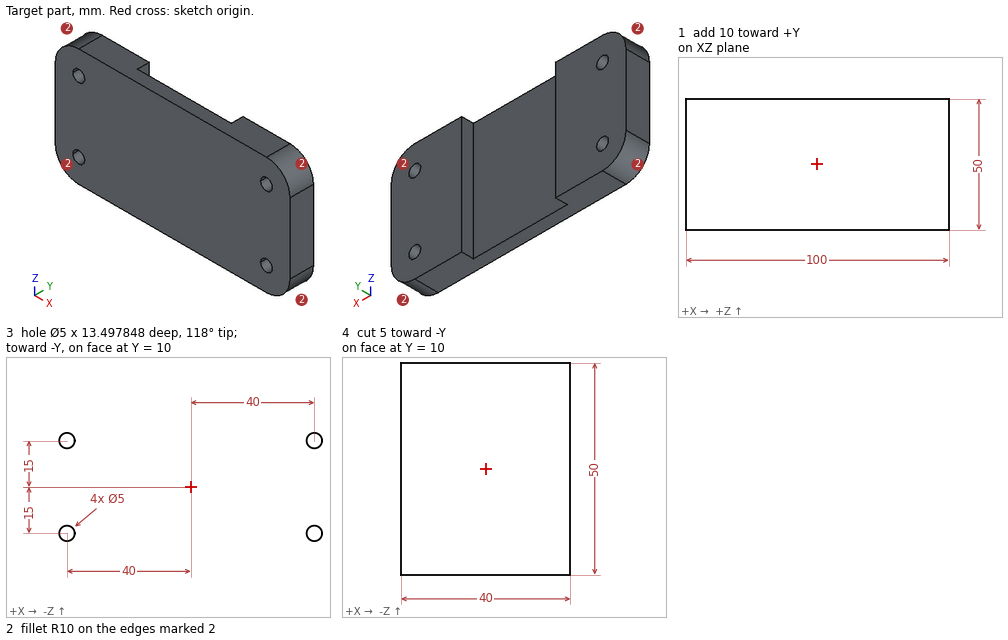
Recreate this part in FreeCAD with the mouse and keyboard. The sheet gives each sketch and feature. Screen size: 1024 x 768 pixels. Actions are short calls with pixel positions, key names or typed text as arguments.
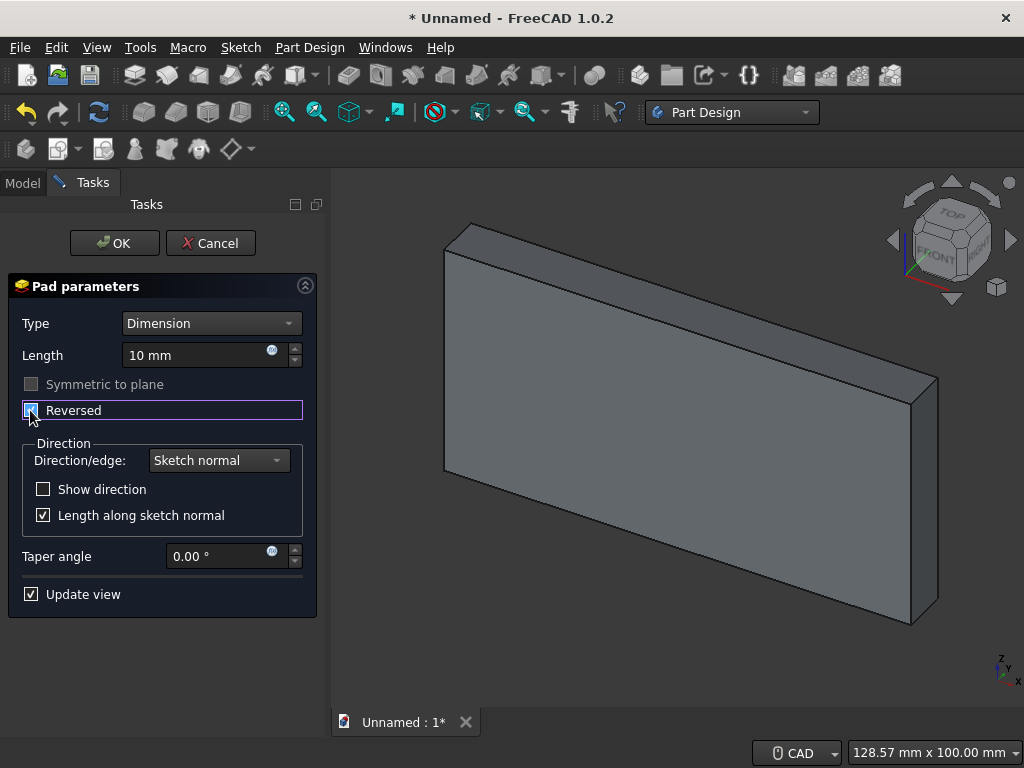
click(115, 243)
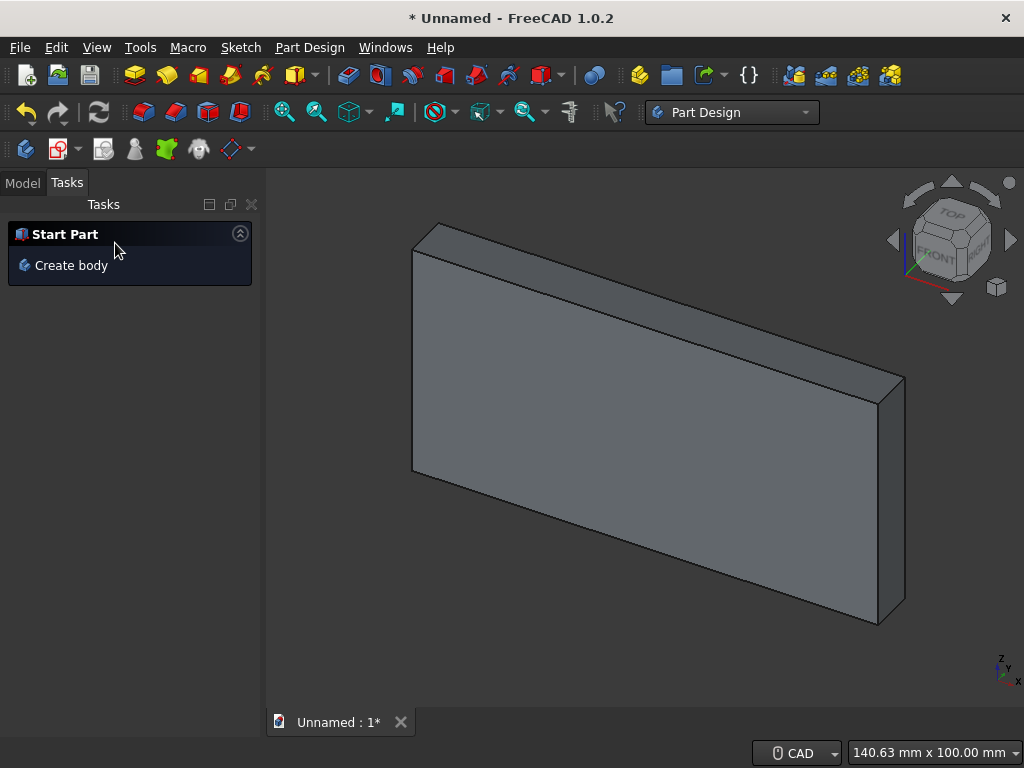
click(892, 390)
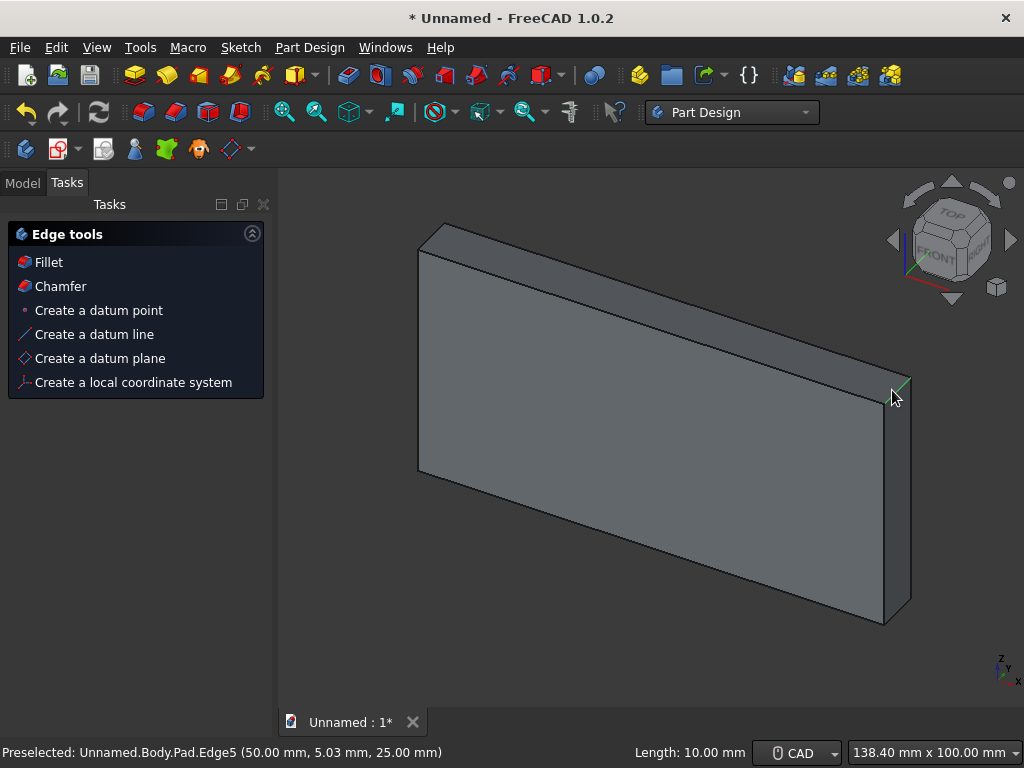
key(0)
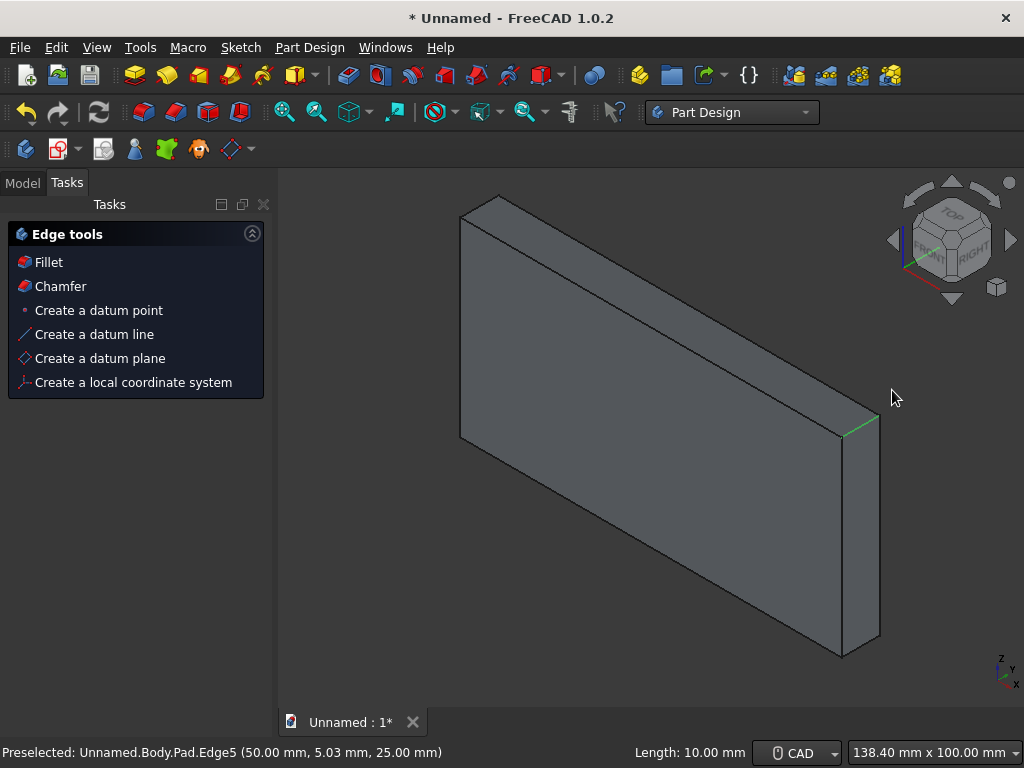
key(2)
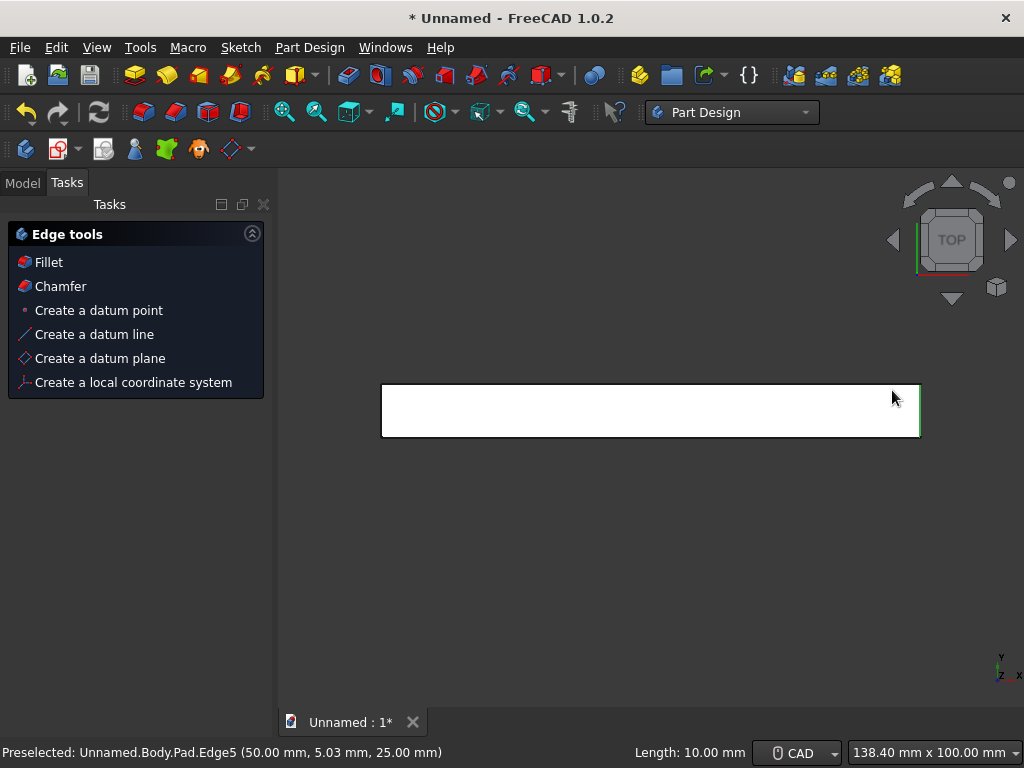
click(381, 410, ctrl)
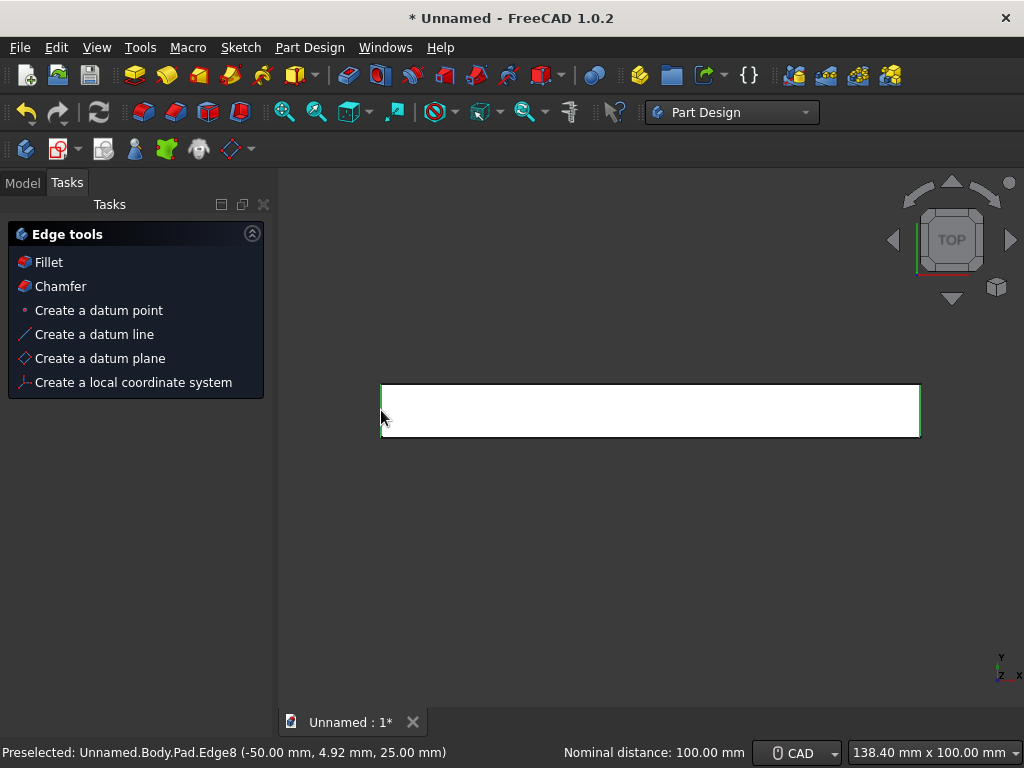
key(1)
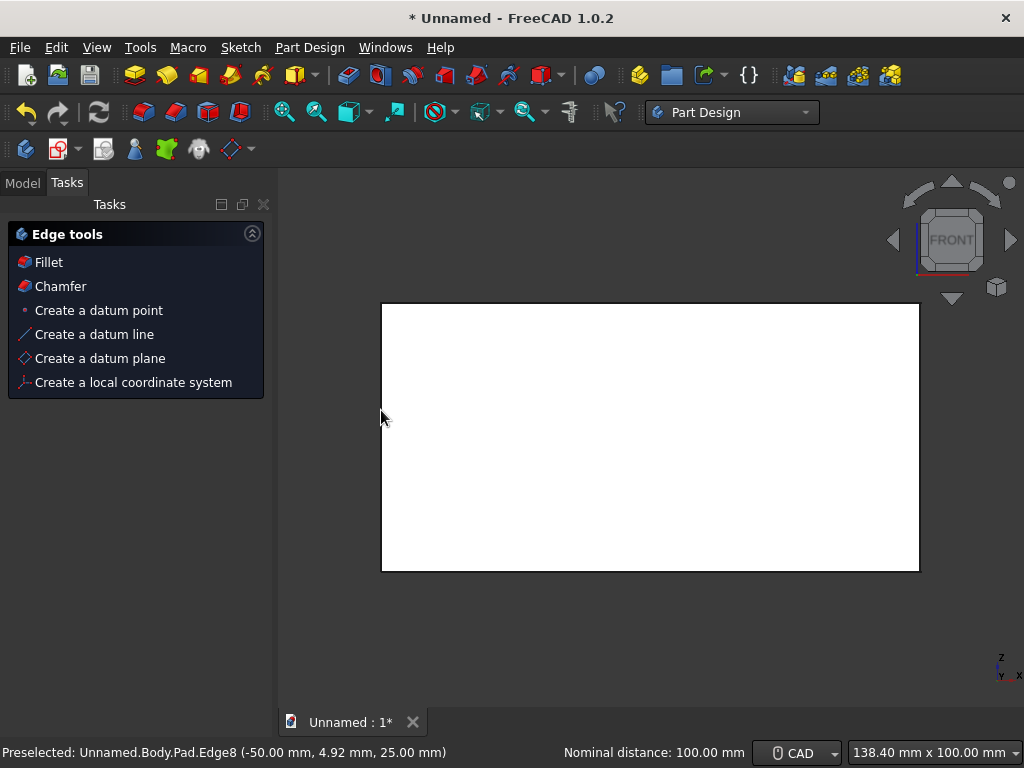
key(3)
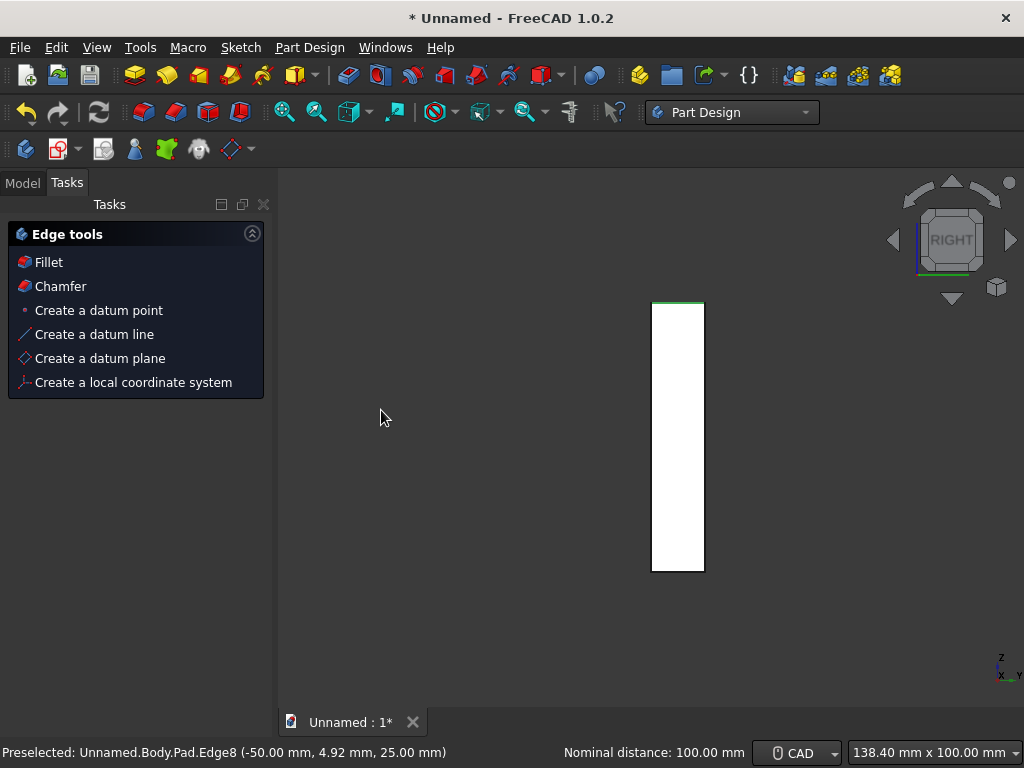
click(678, 571, ctrl)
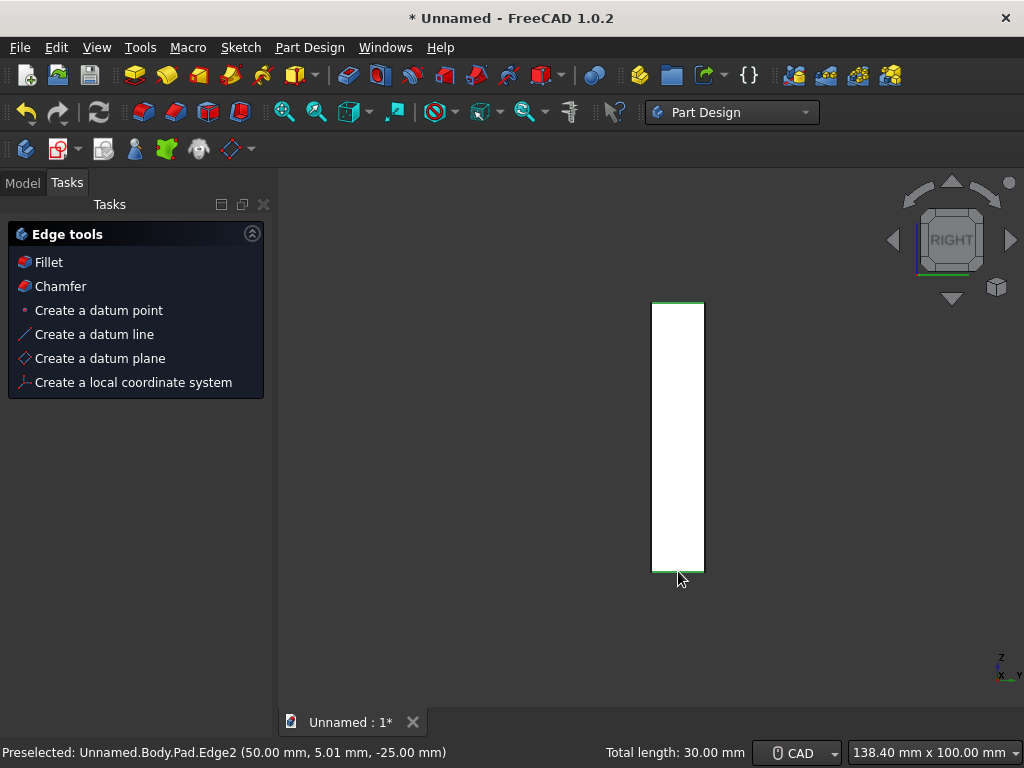
key(5)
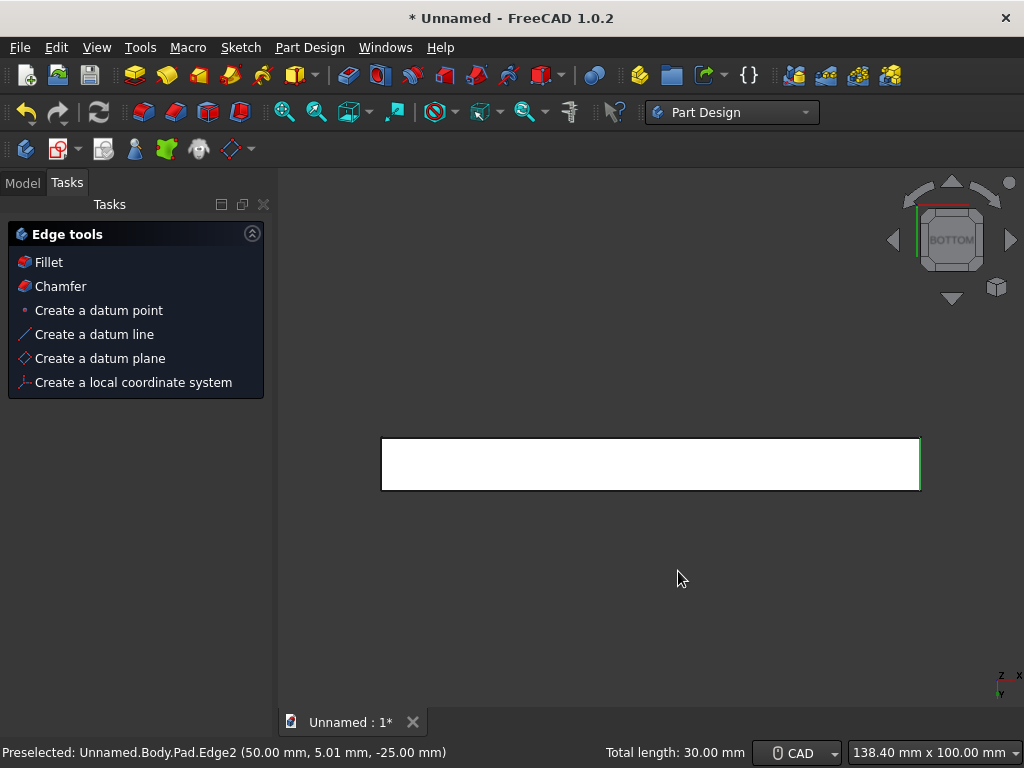
click(382, 463, ctrl)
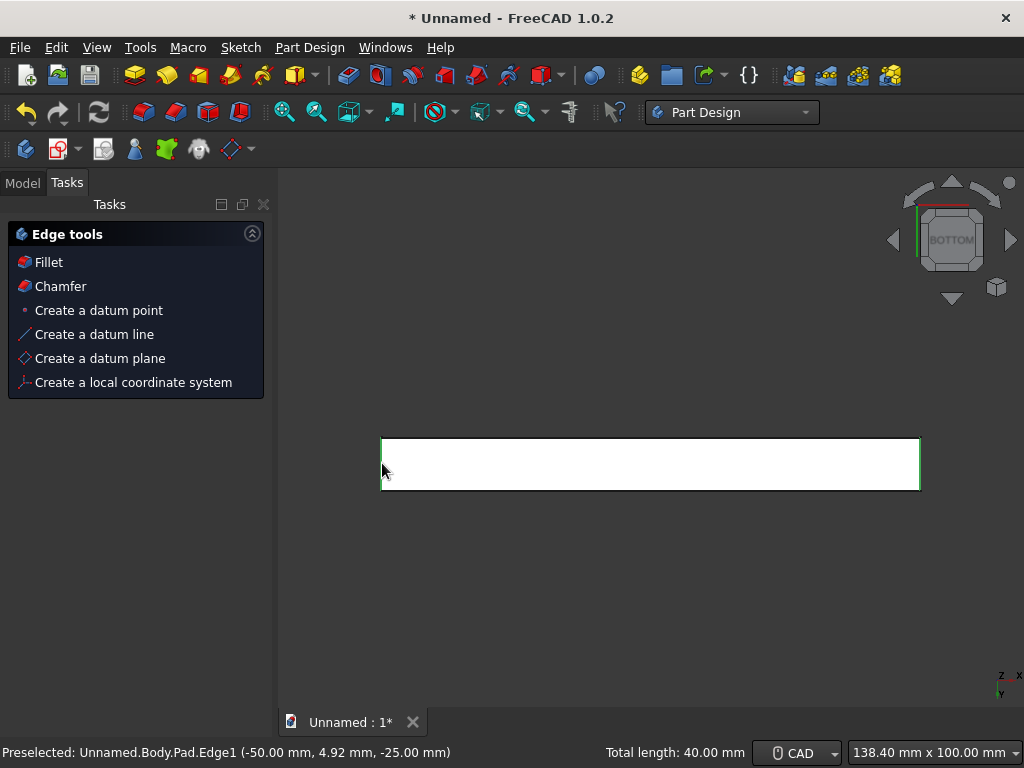
click(144, 112)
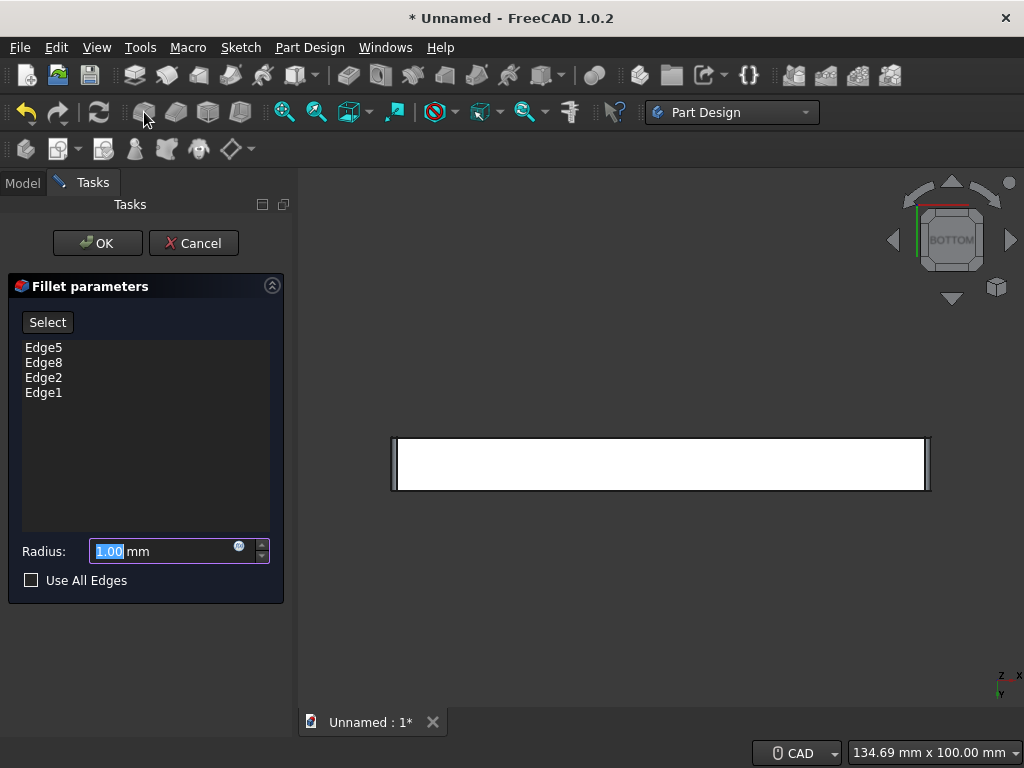
text(10)
key(Tab)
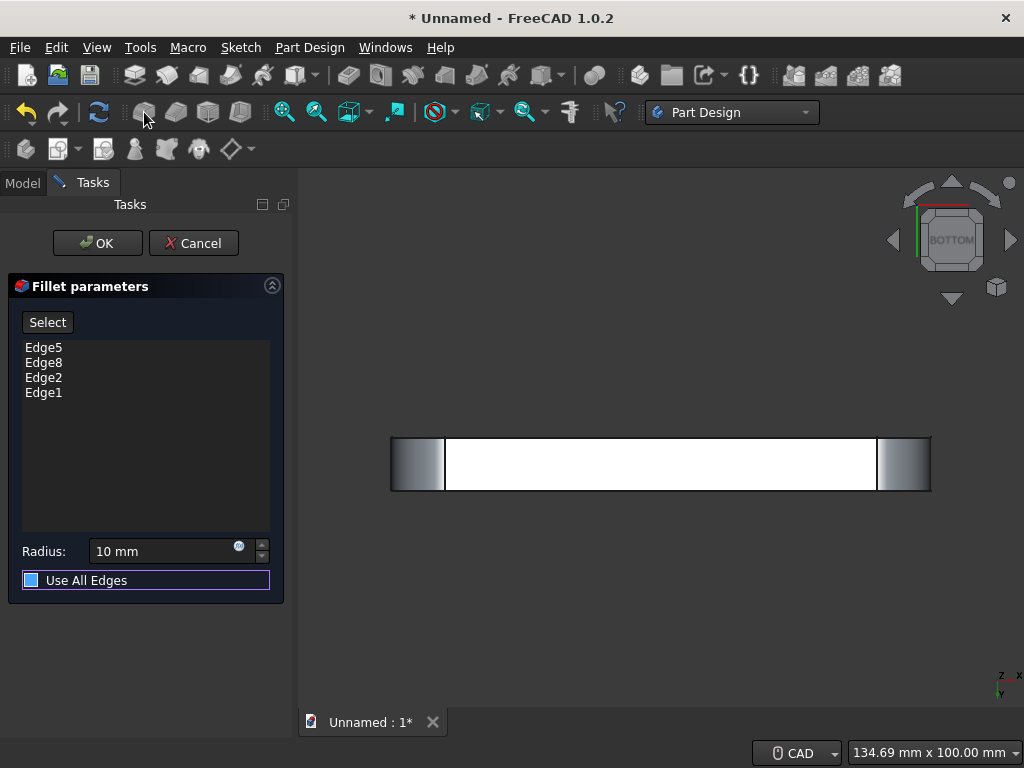
click(98, 243)